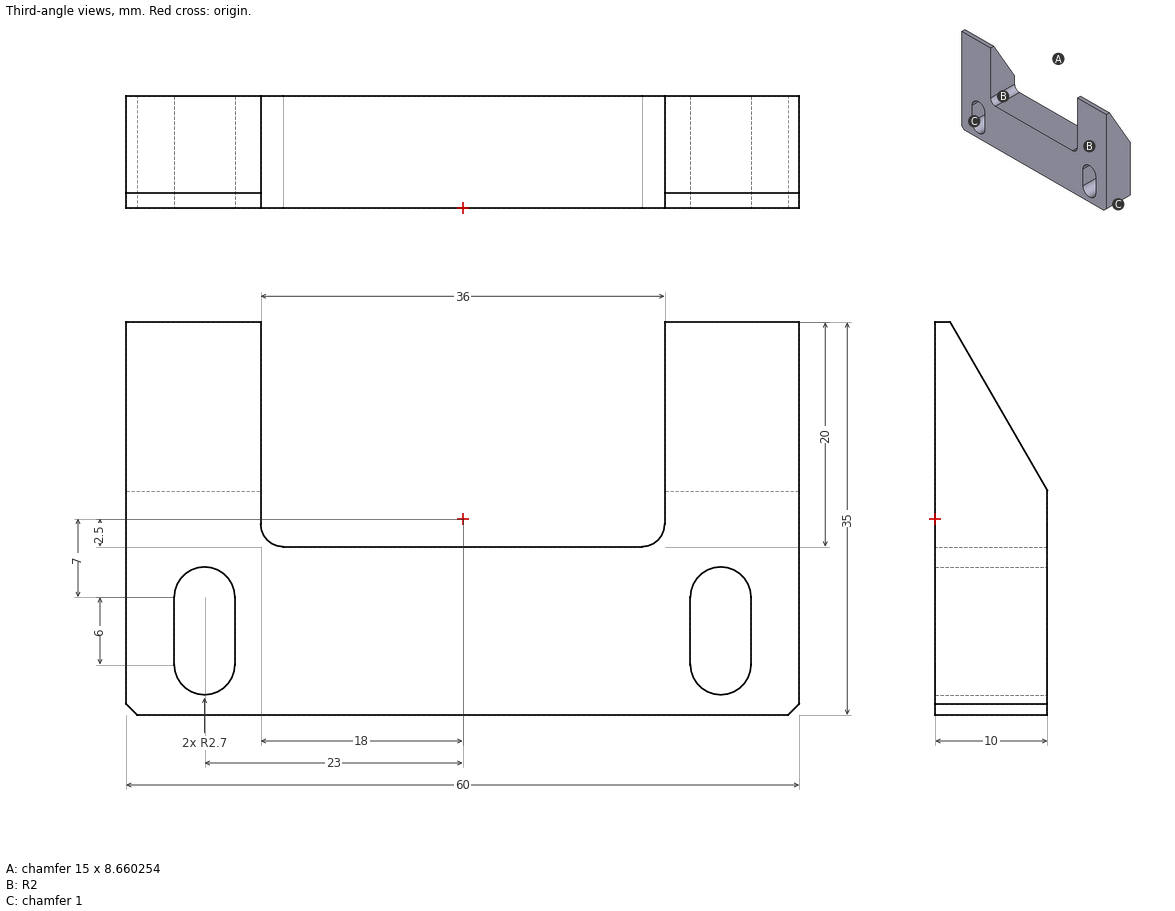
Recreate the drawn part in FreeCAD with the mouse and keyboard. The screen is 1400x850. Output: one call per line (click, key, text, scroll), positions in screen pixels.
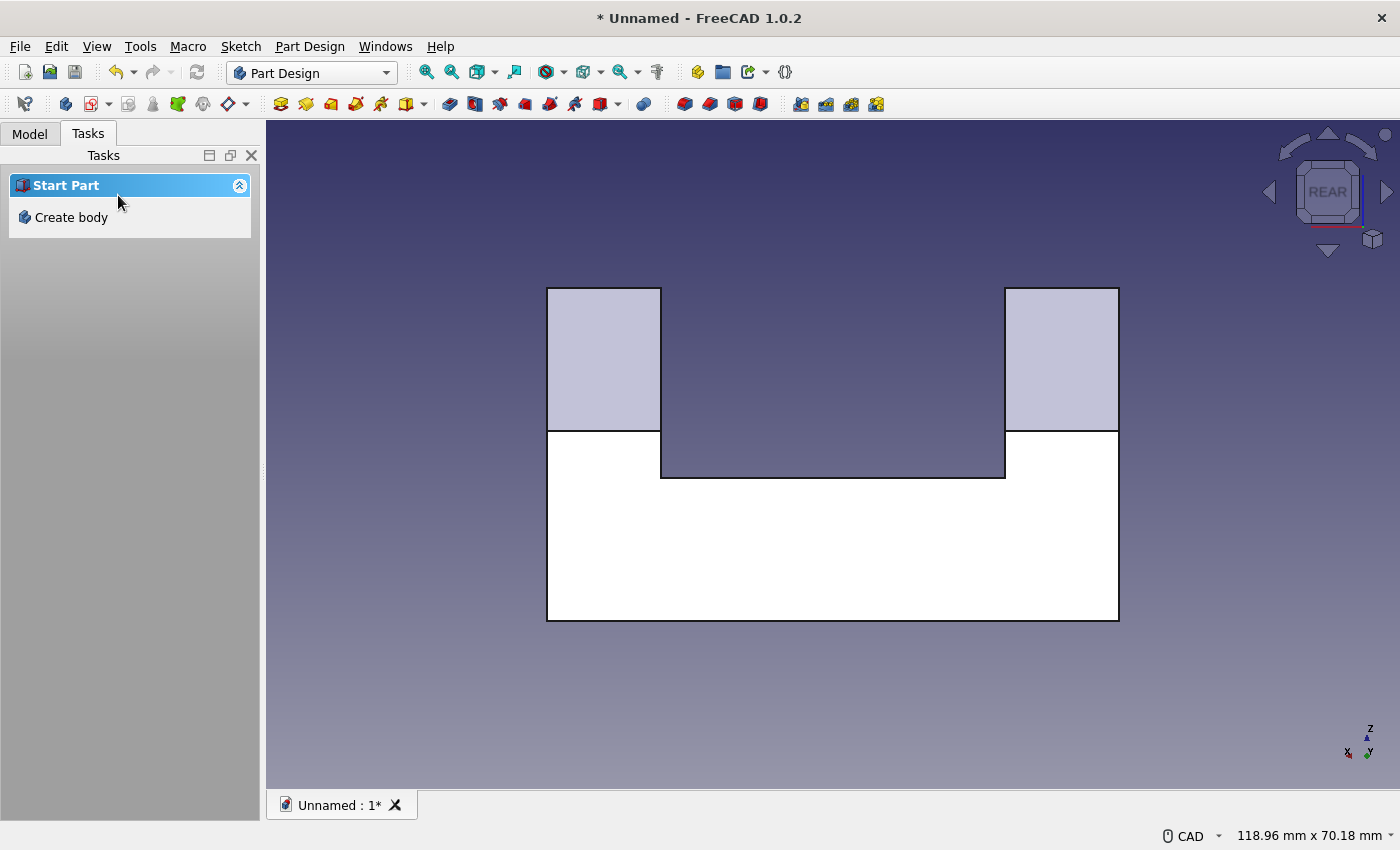
key(6)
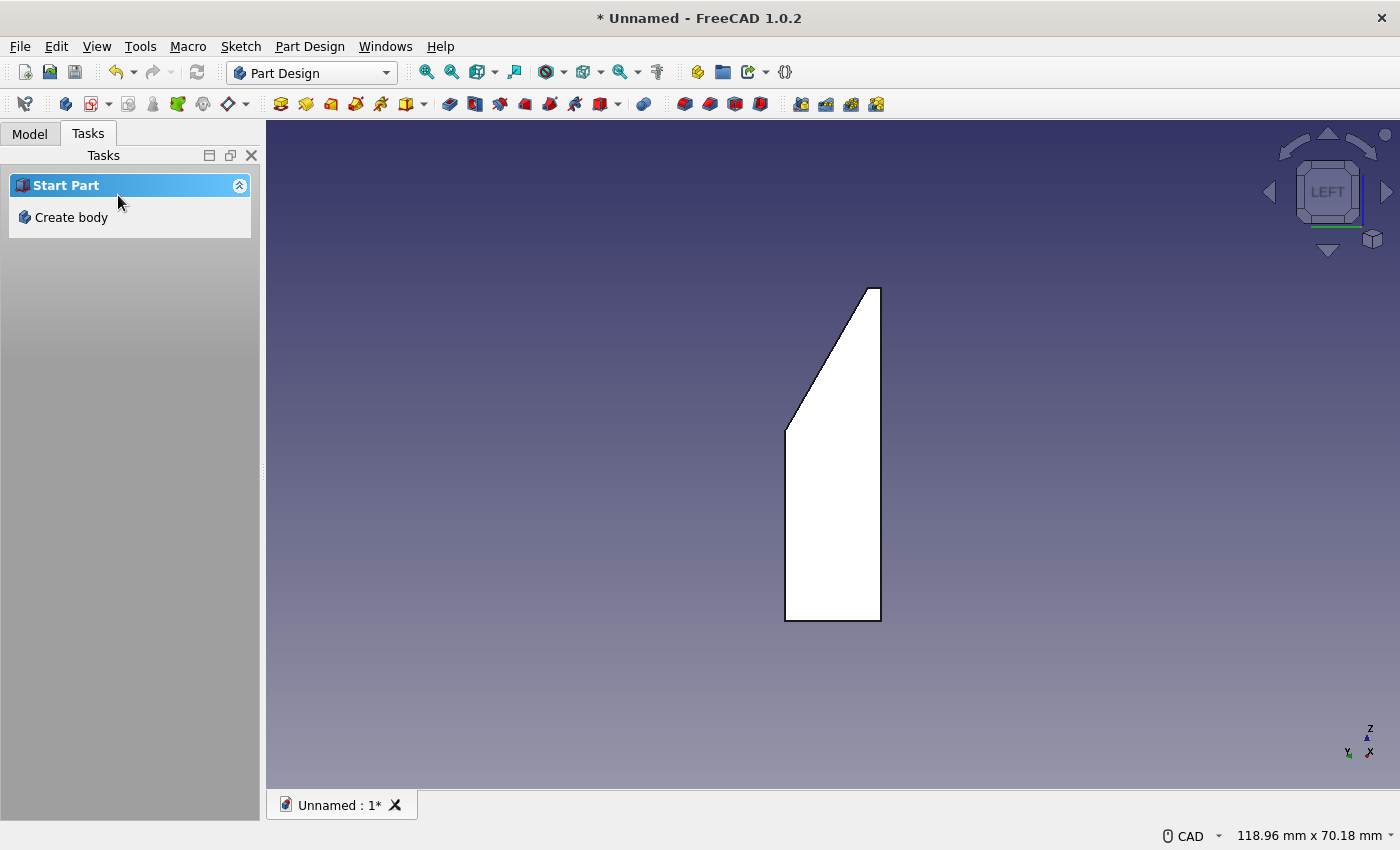
key(v)
key(3)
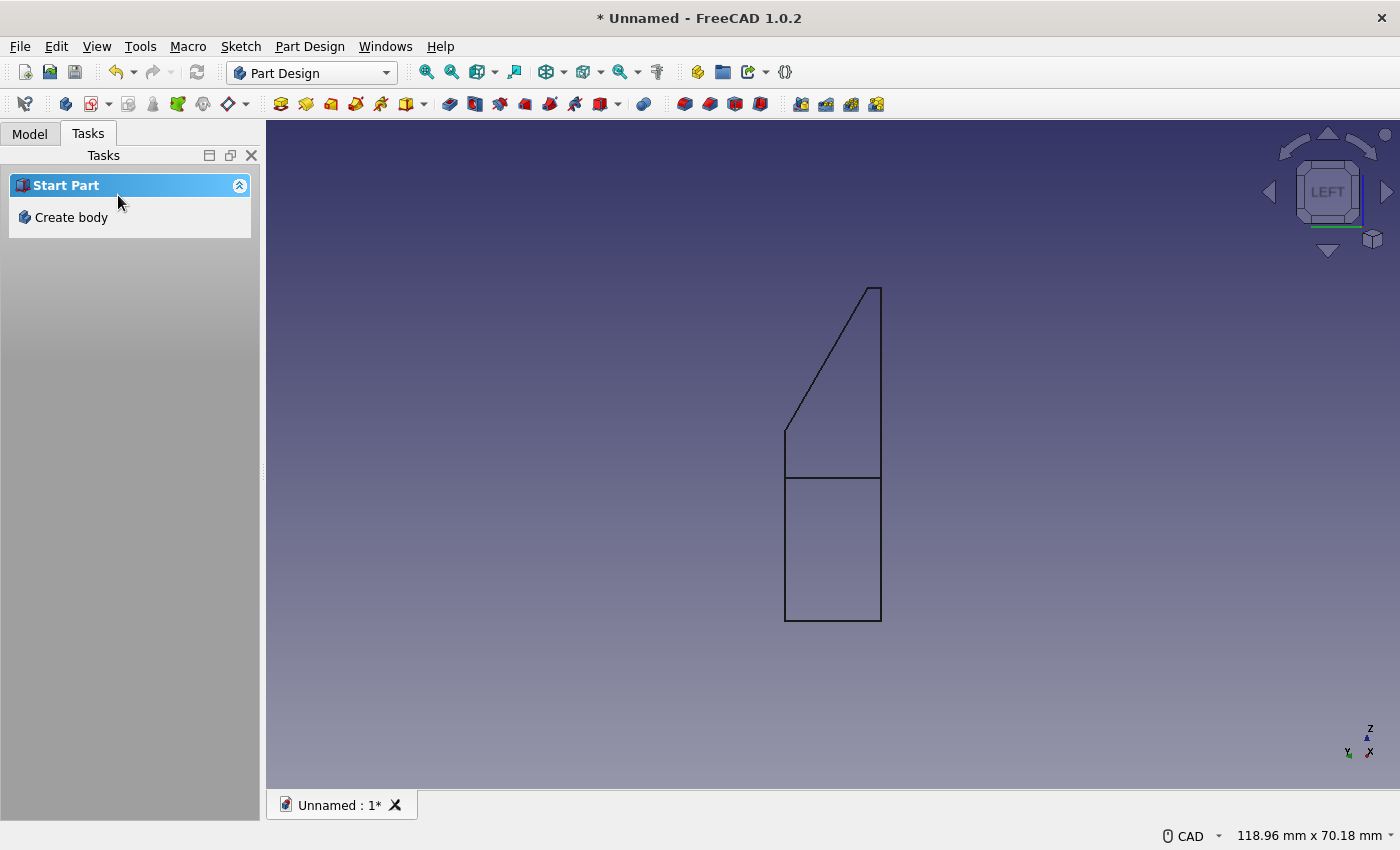
key(0)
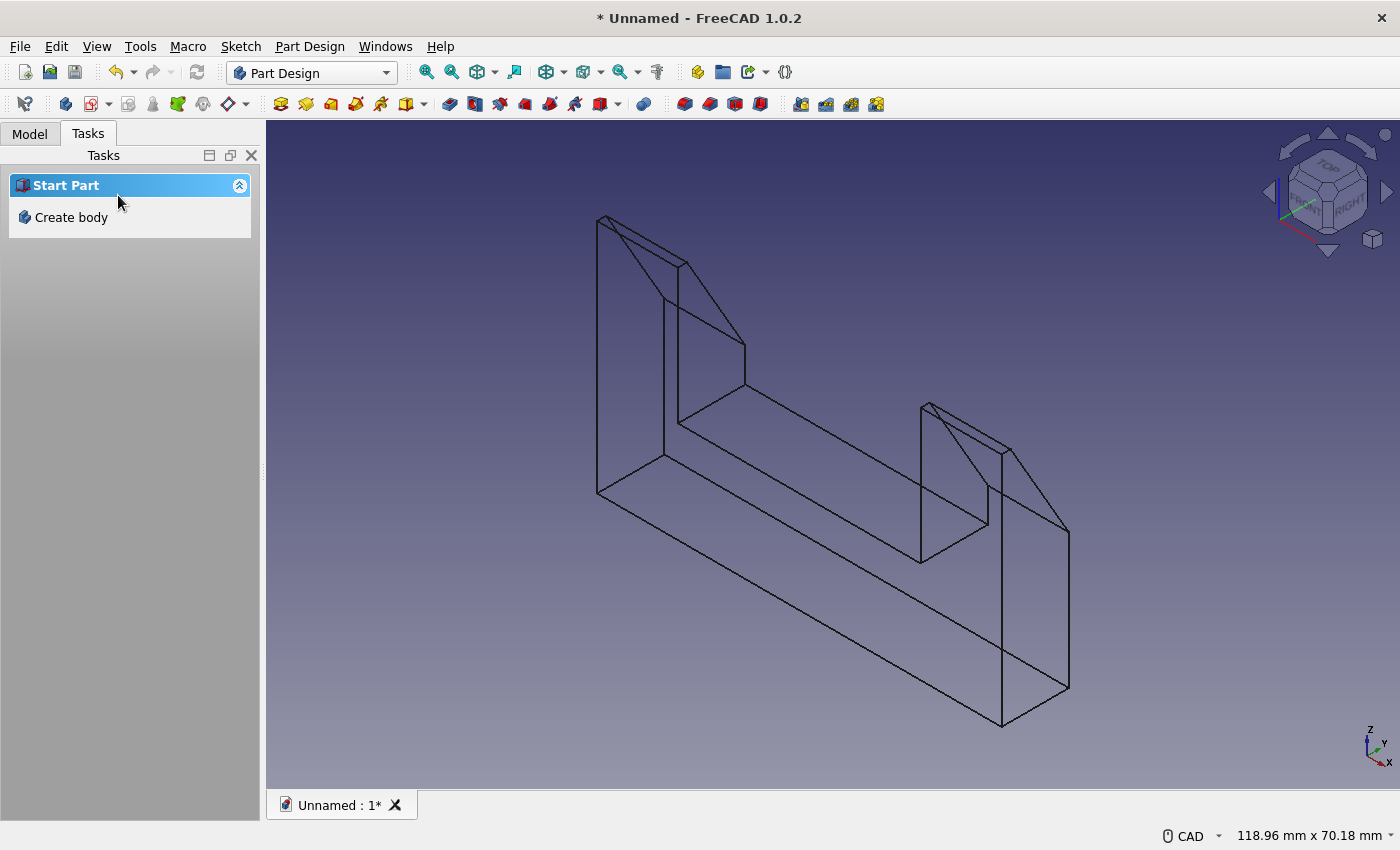
click(712, 403)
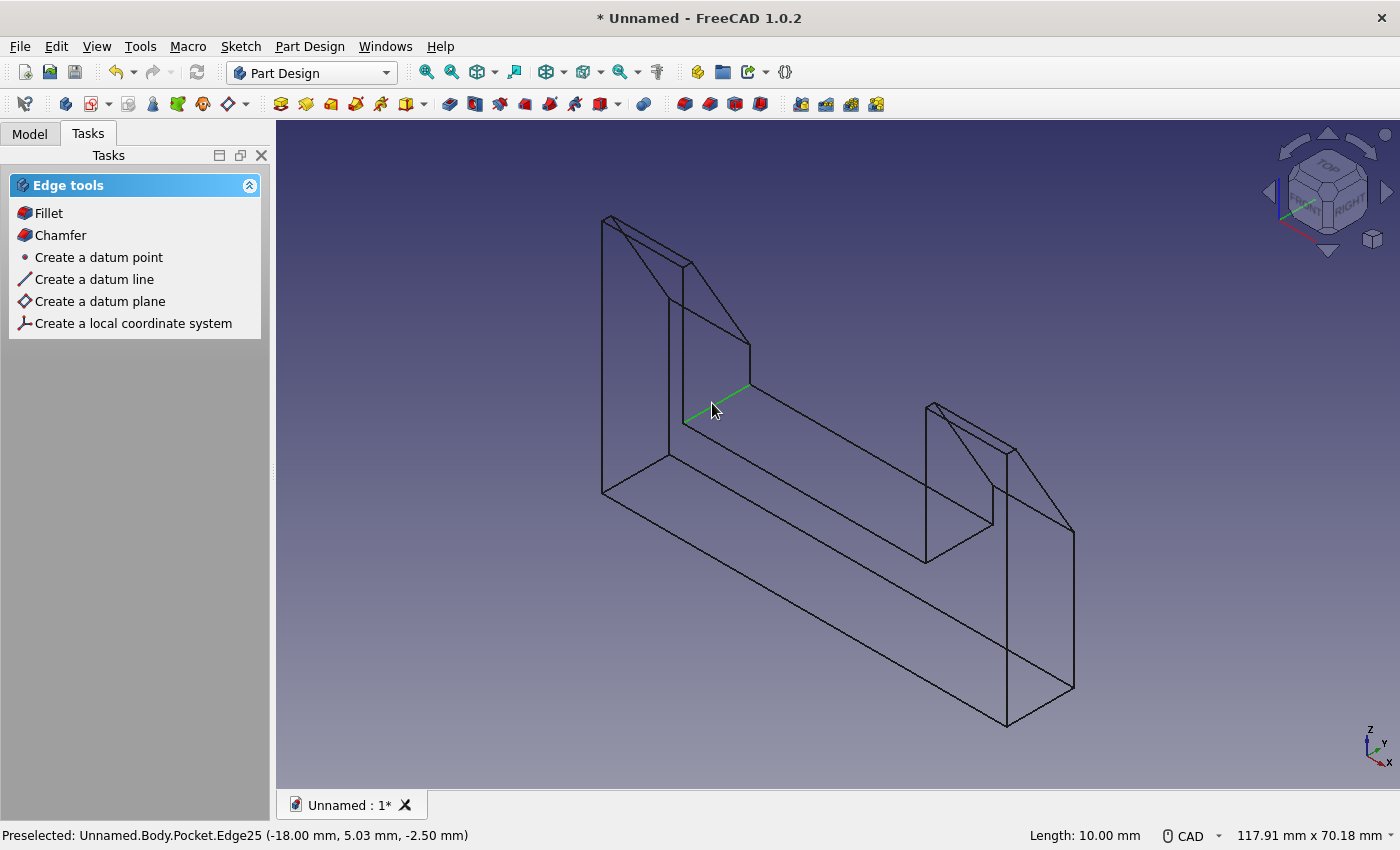
click(959, 543, ctrl)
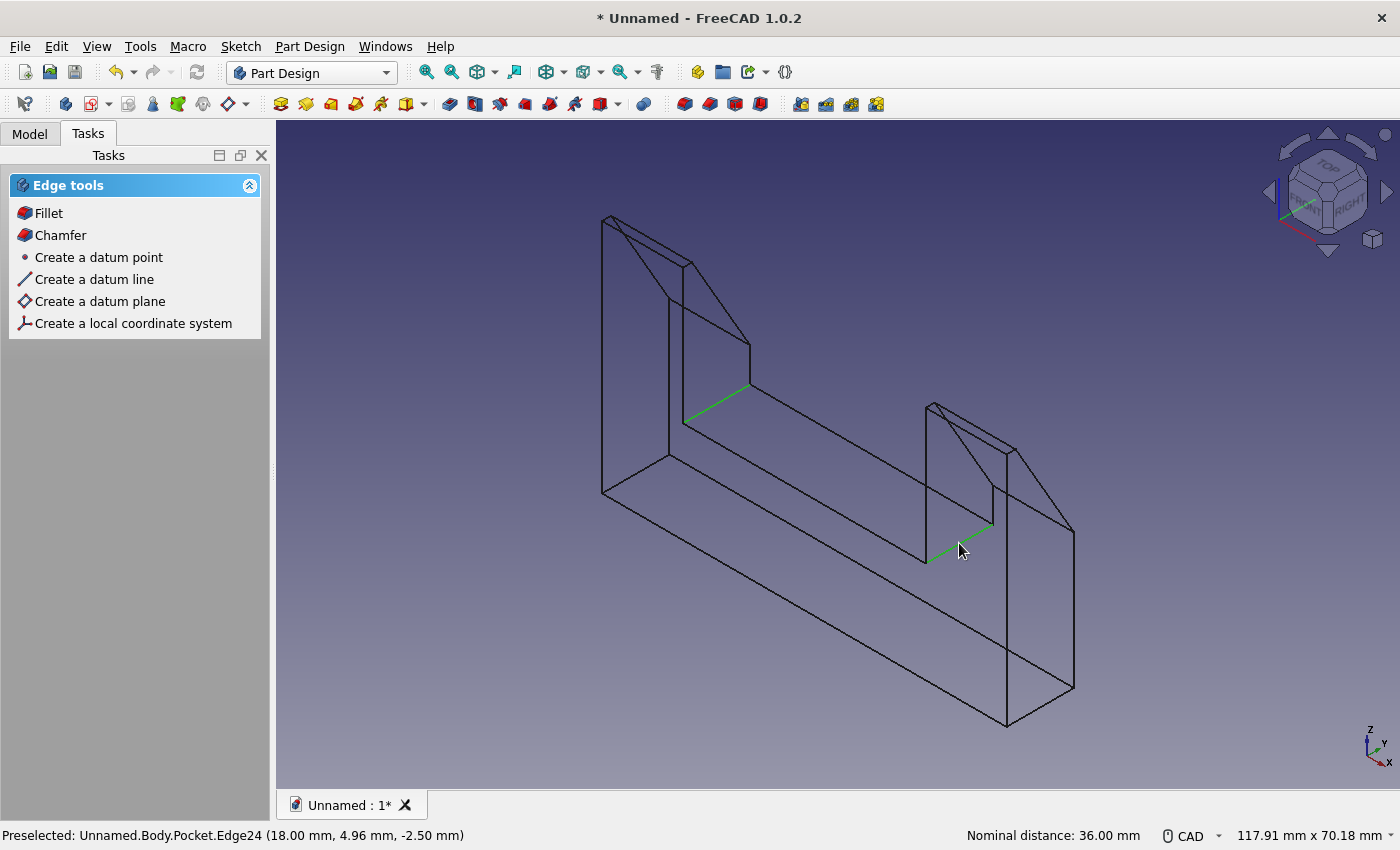
key(v)
key(1)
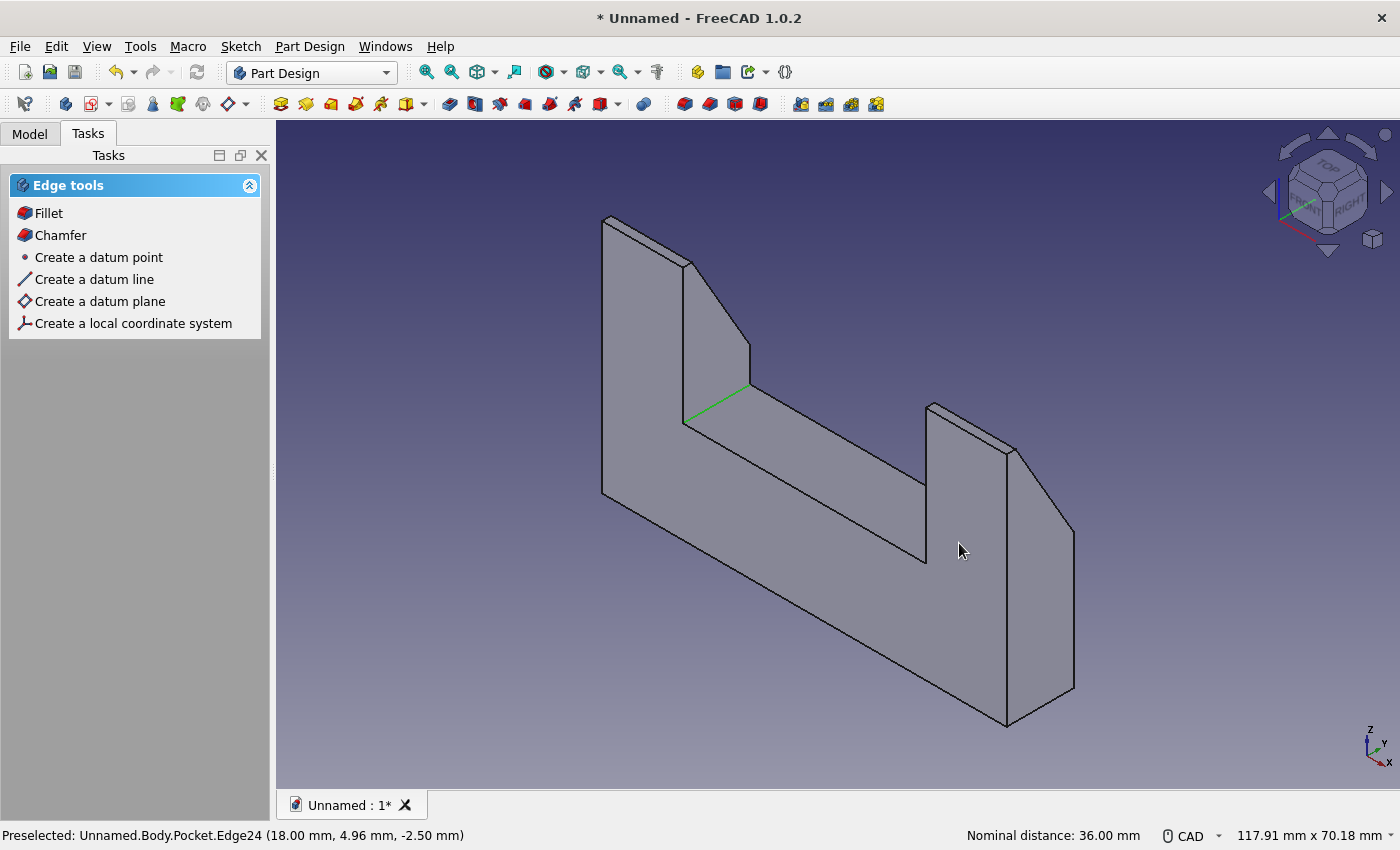
click(685, 104)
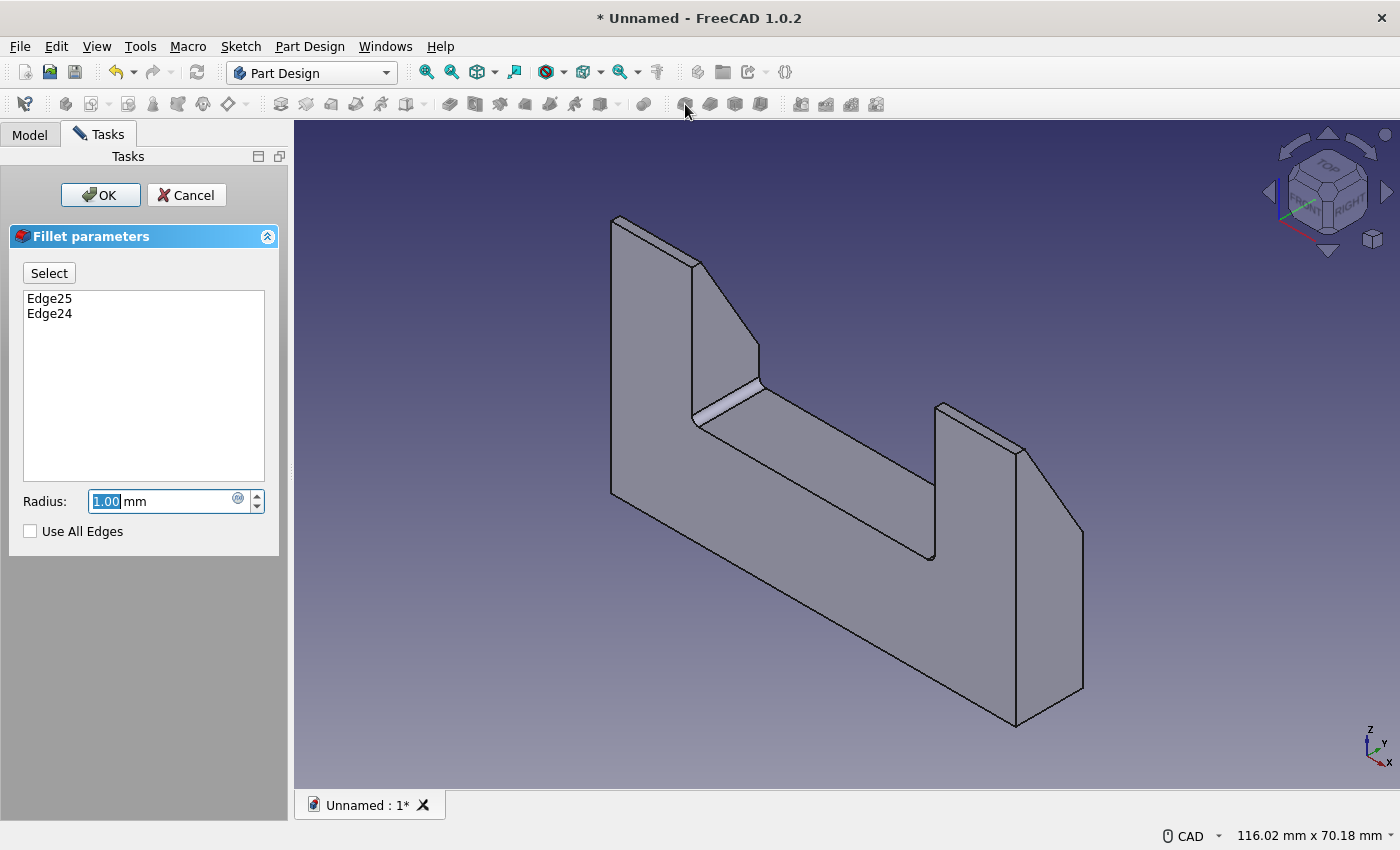
text(2)
key(Tab)